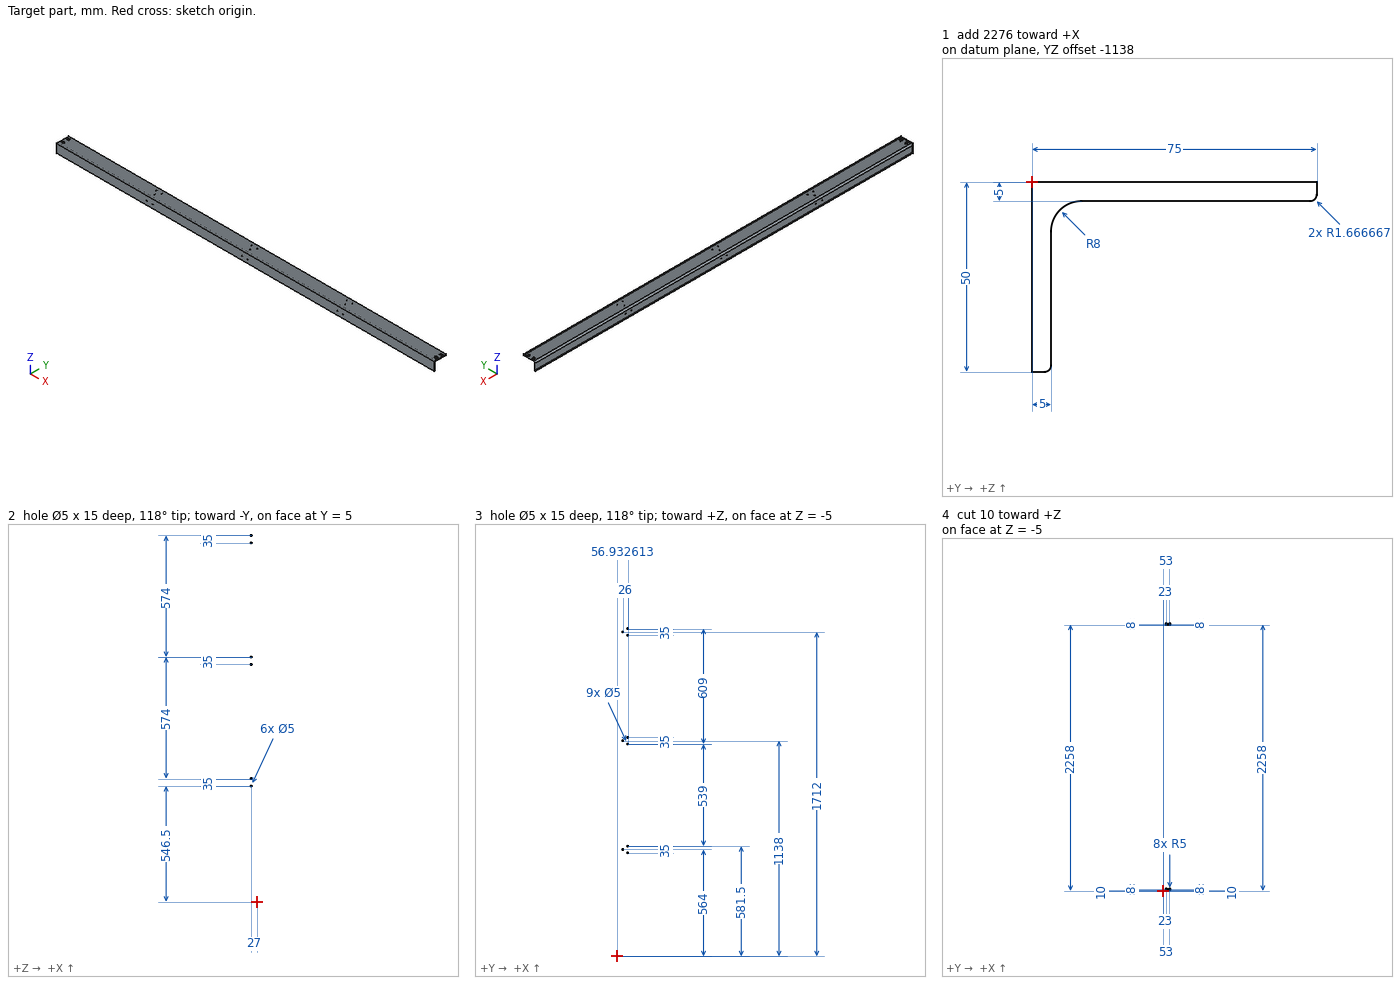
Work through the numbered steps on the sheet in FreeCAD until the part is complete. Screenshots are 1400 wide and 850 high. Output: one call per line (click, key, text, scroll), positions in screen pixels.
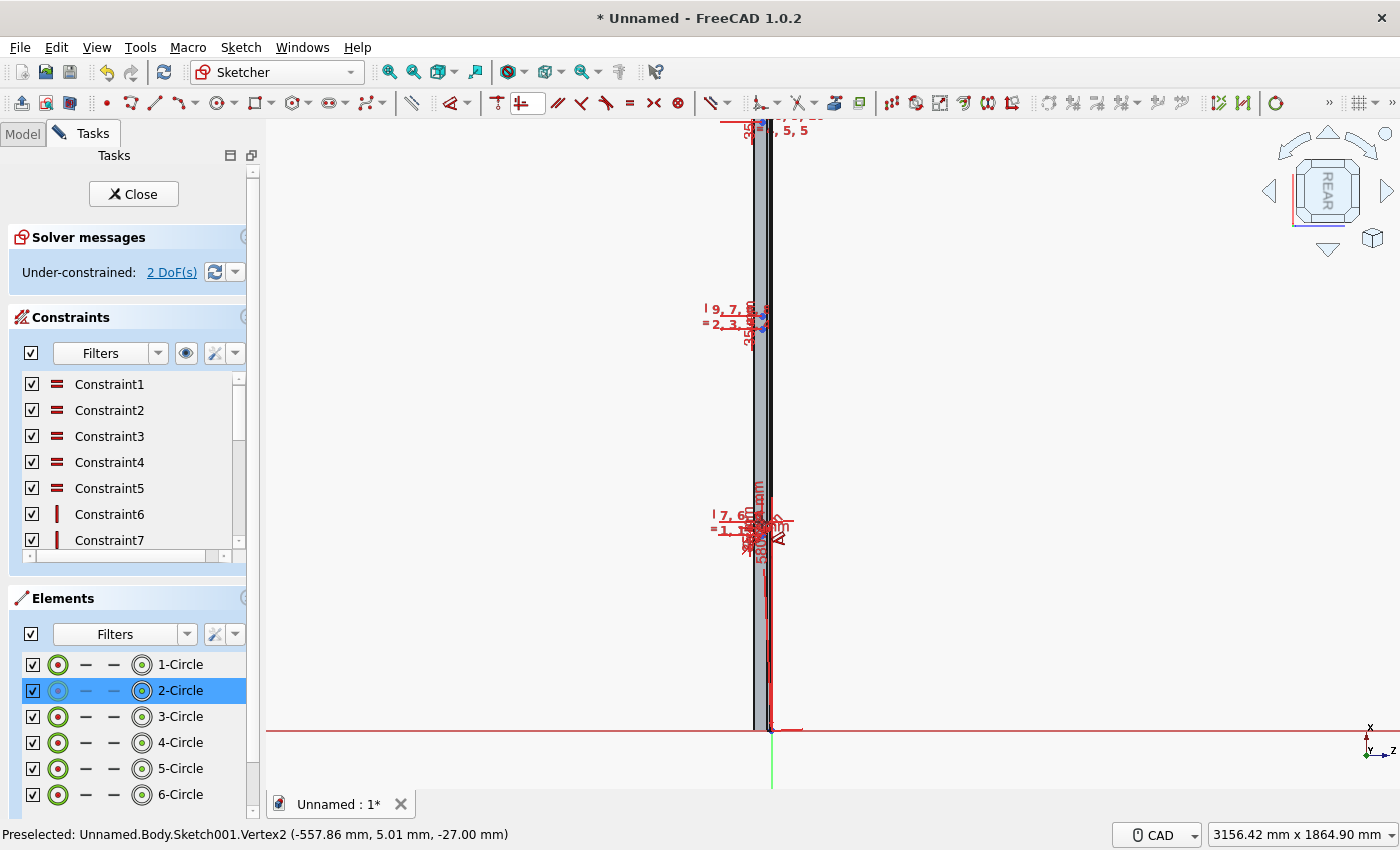
click(762, 316)
click(728, 419)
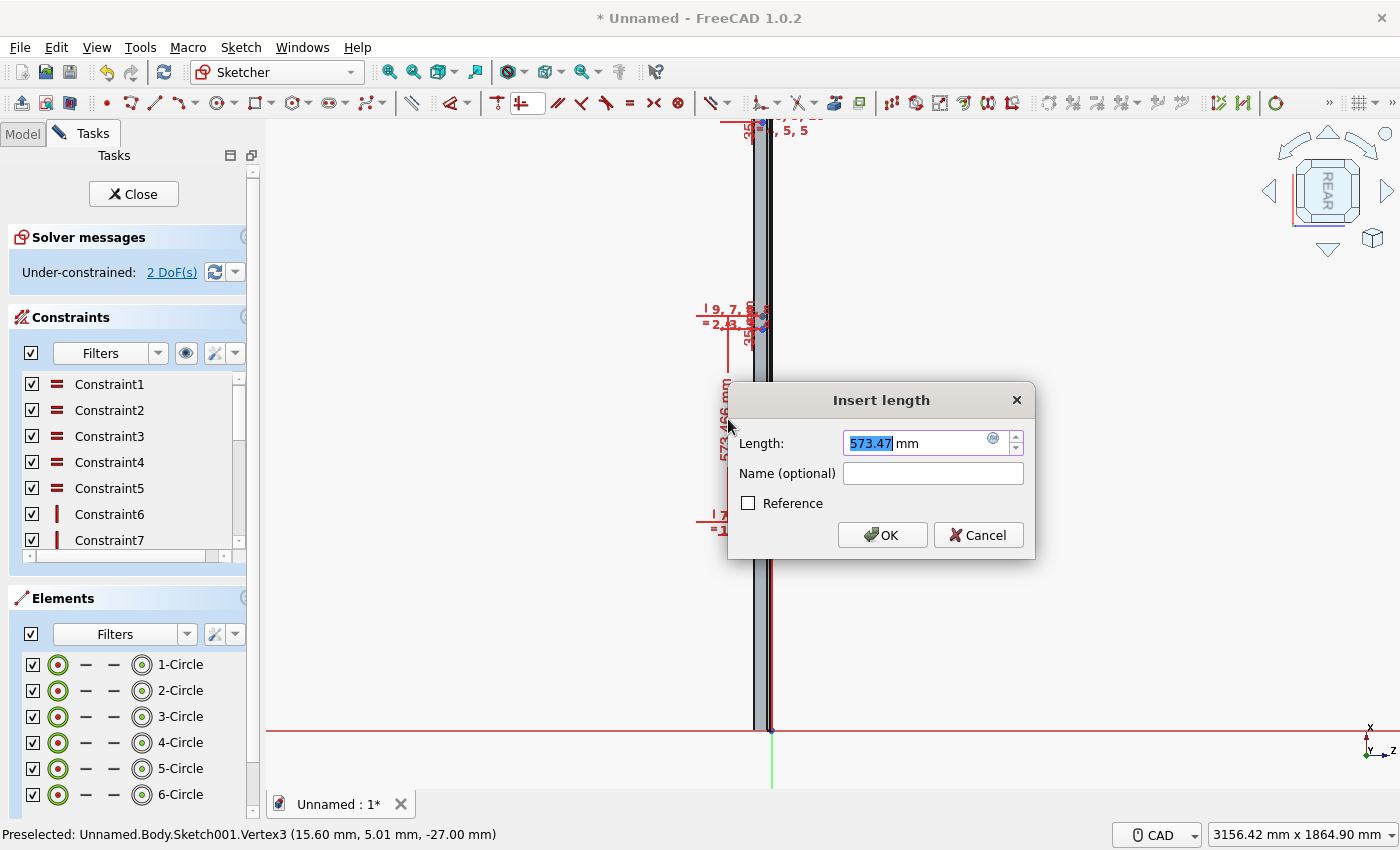
text(574)
key(Return)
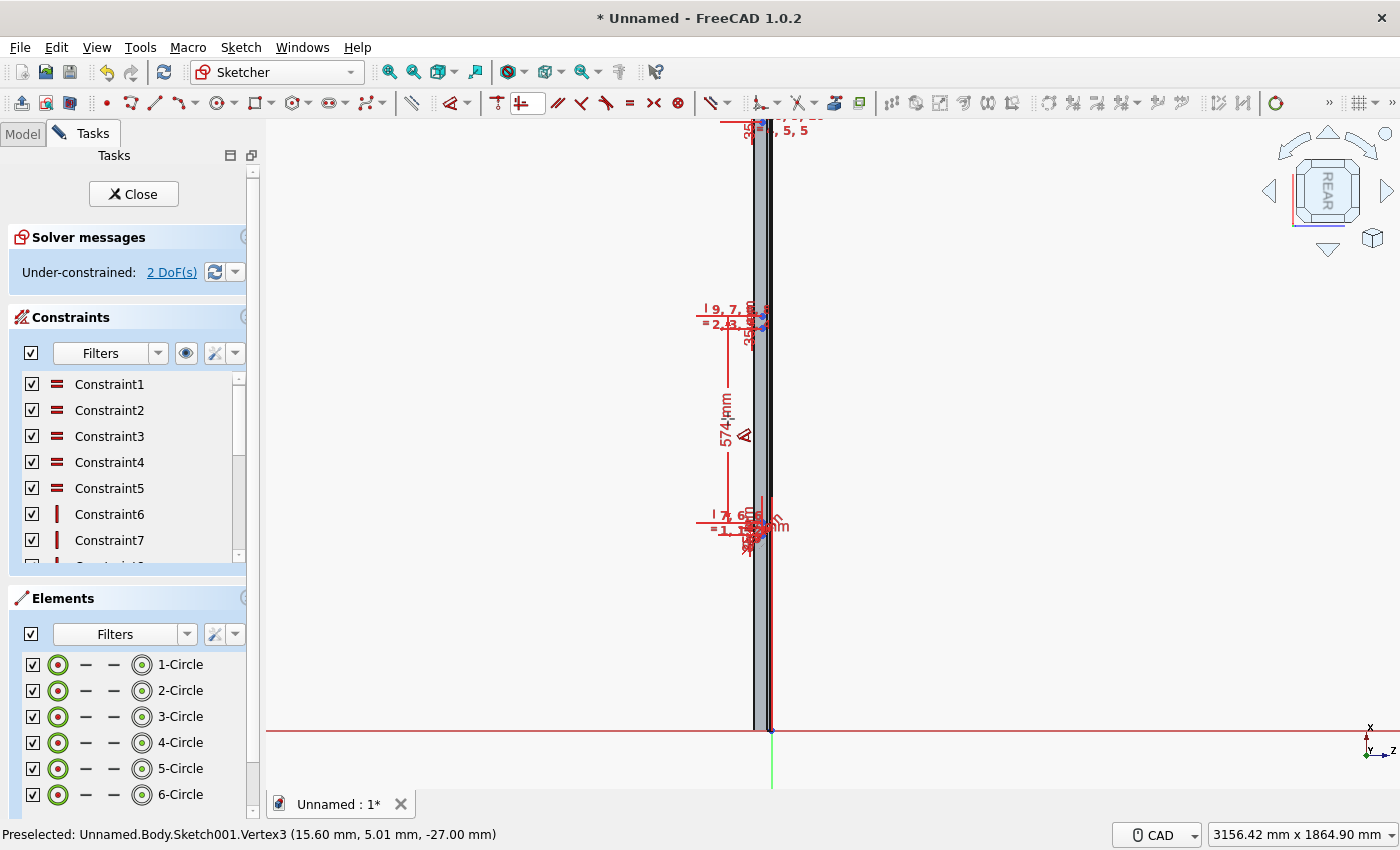
click(762, 316)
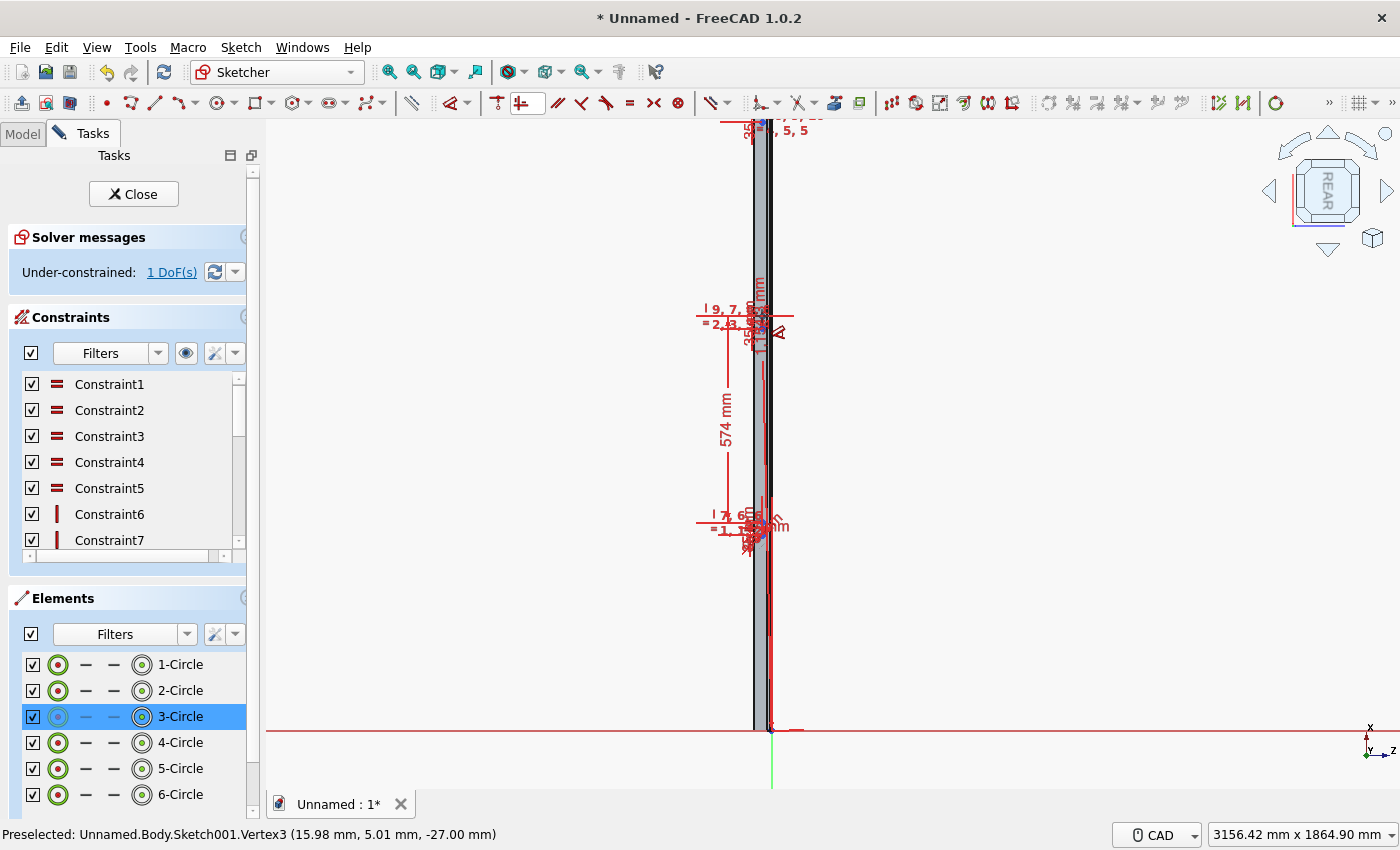
scroll(761, 524, down, 2)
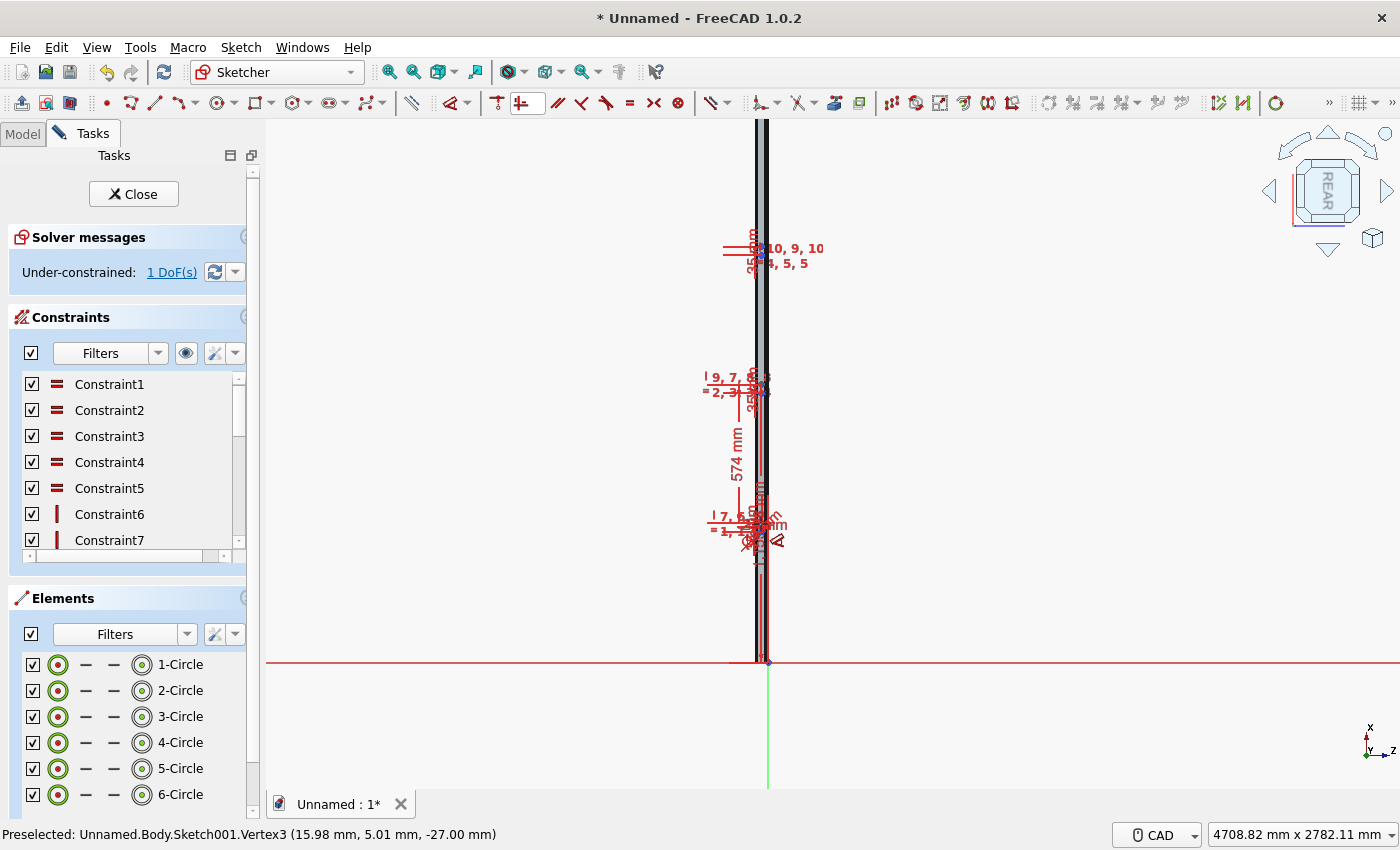
scroll(762, 247, up, 2)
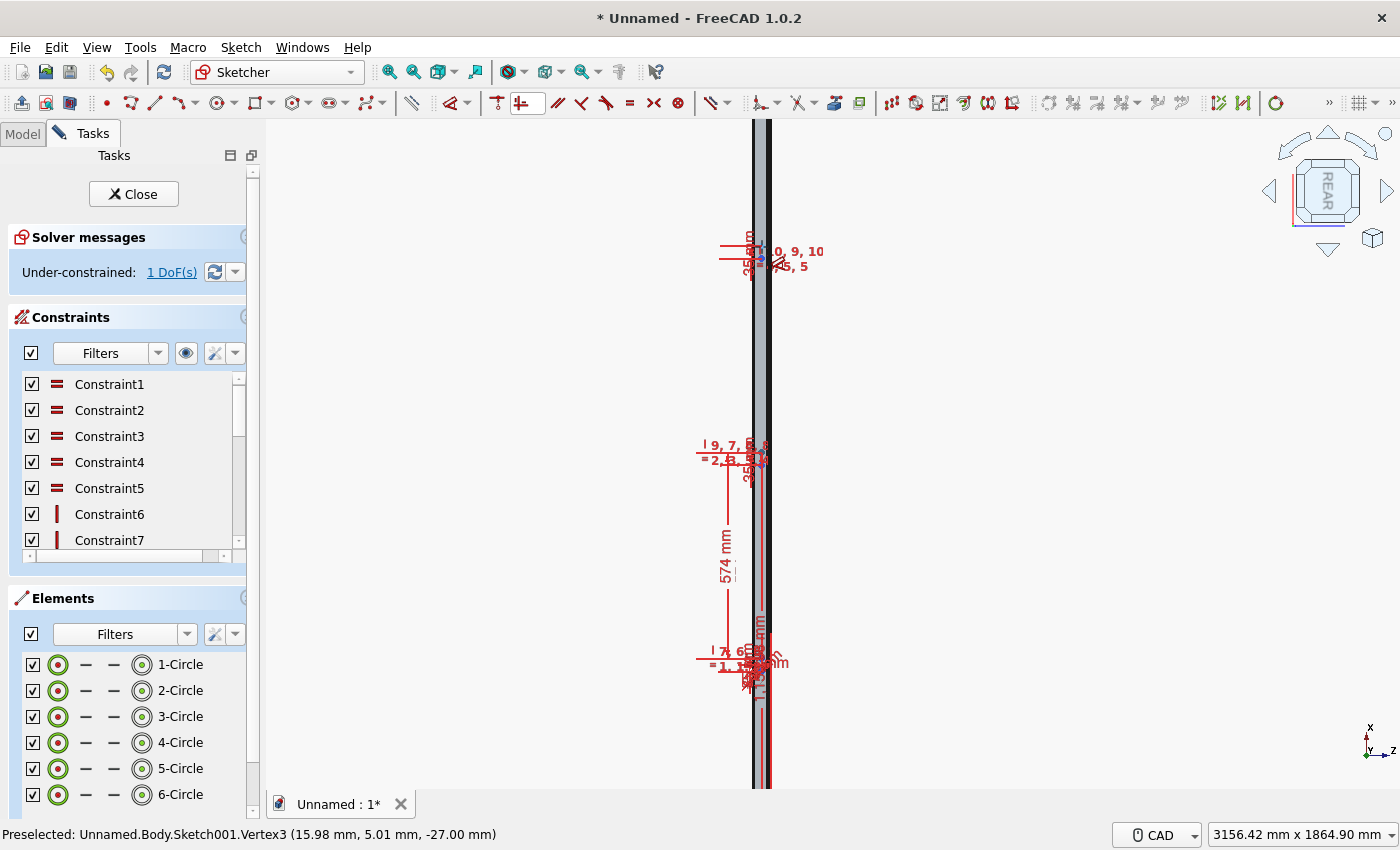
click(762, 246)
click(728, 350)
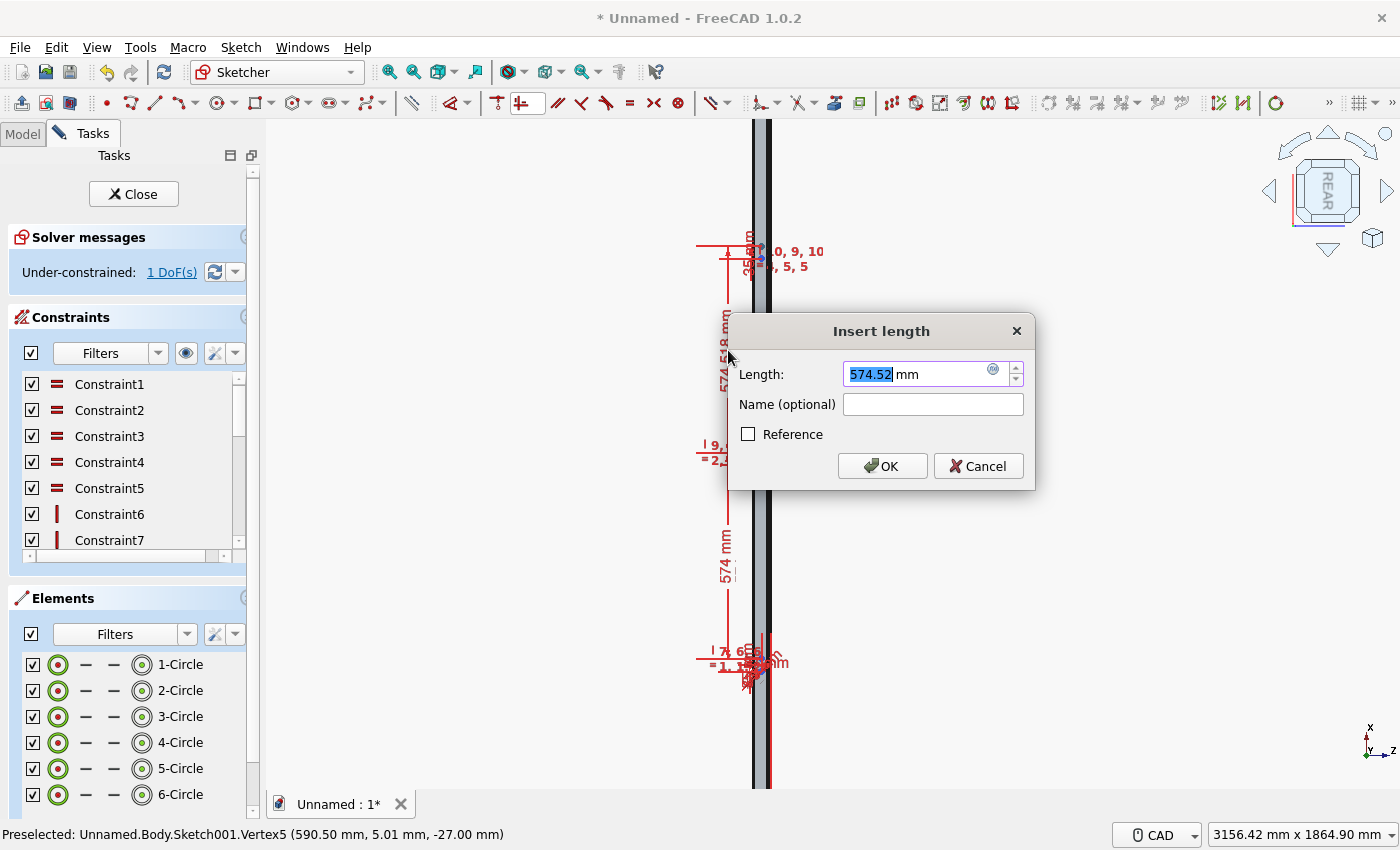
text(574)
key(Return)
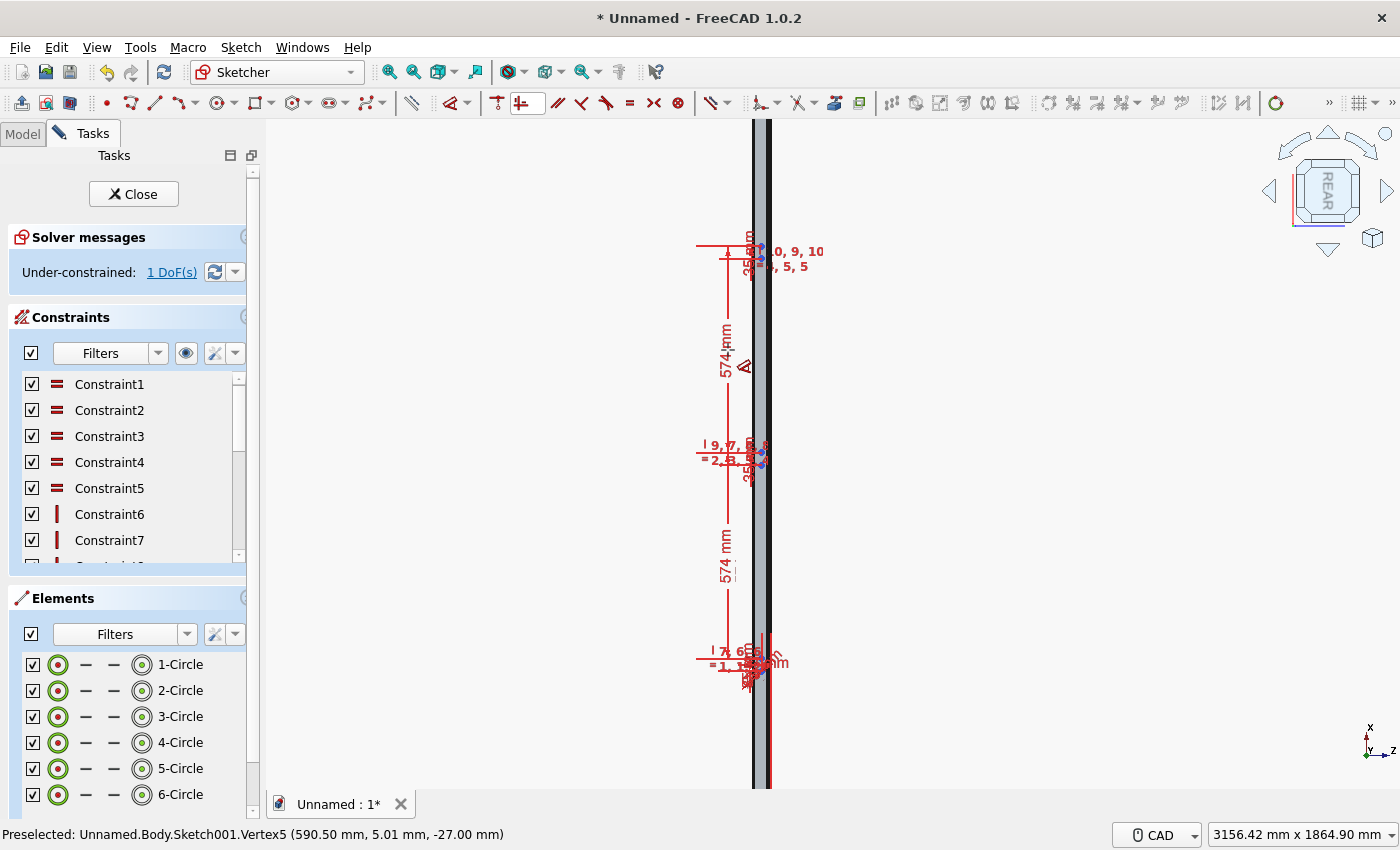
click(762, 671)
click(805, 716)